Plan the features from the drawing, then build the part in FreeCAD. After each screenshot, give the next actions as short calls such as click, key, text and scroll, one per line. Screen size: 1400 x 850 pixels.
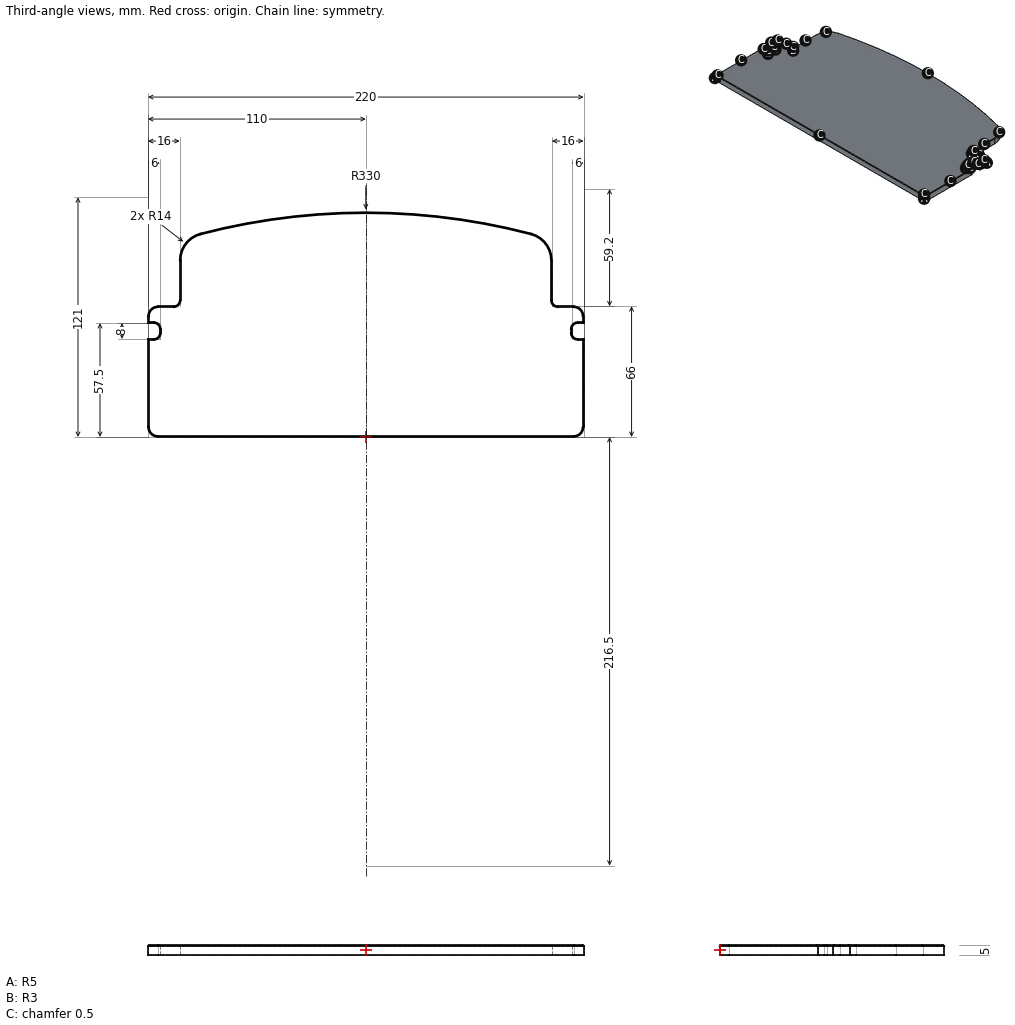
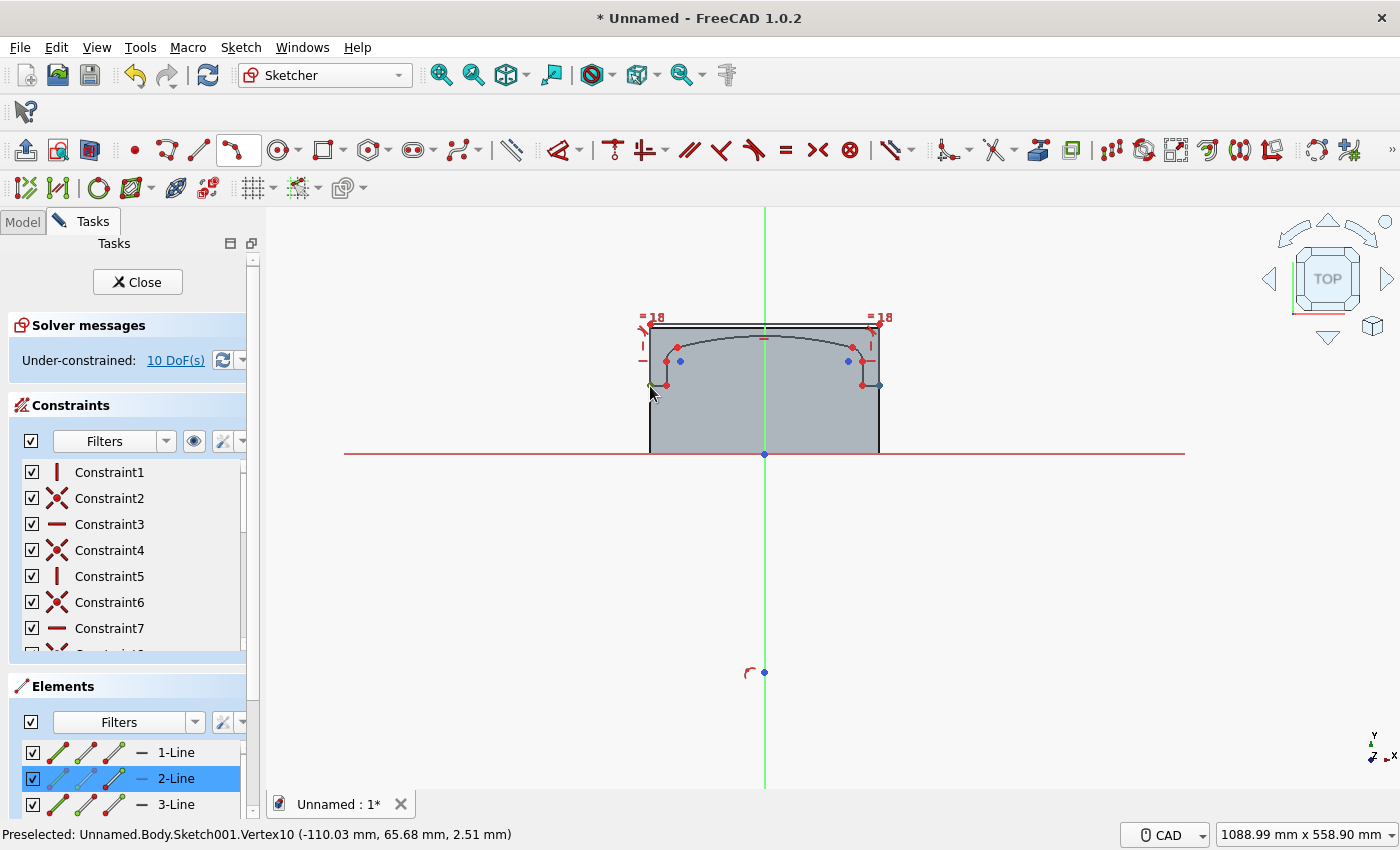
click(765, 723)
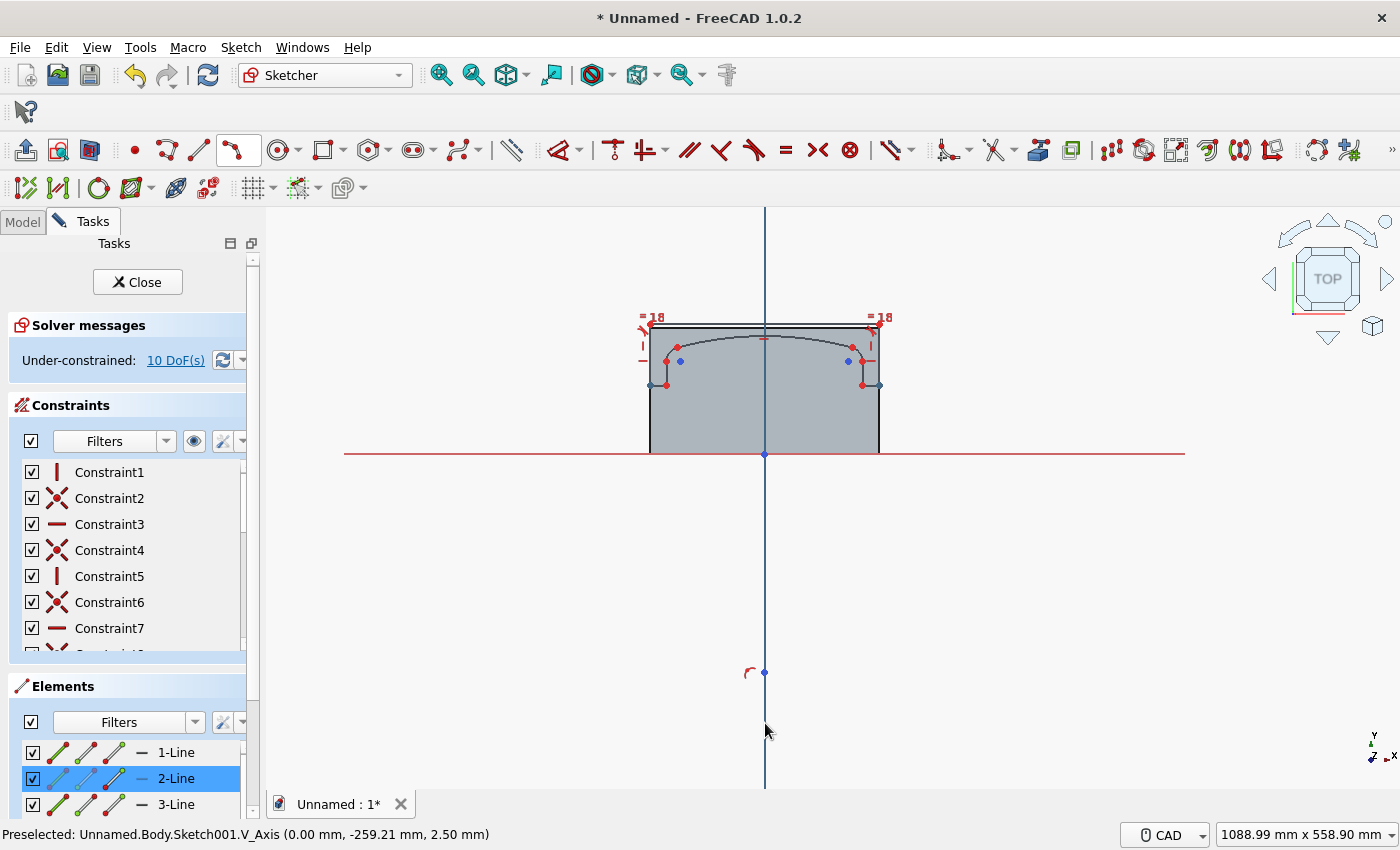
key(s)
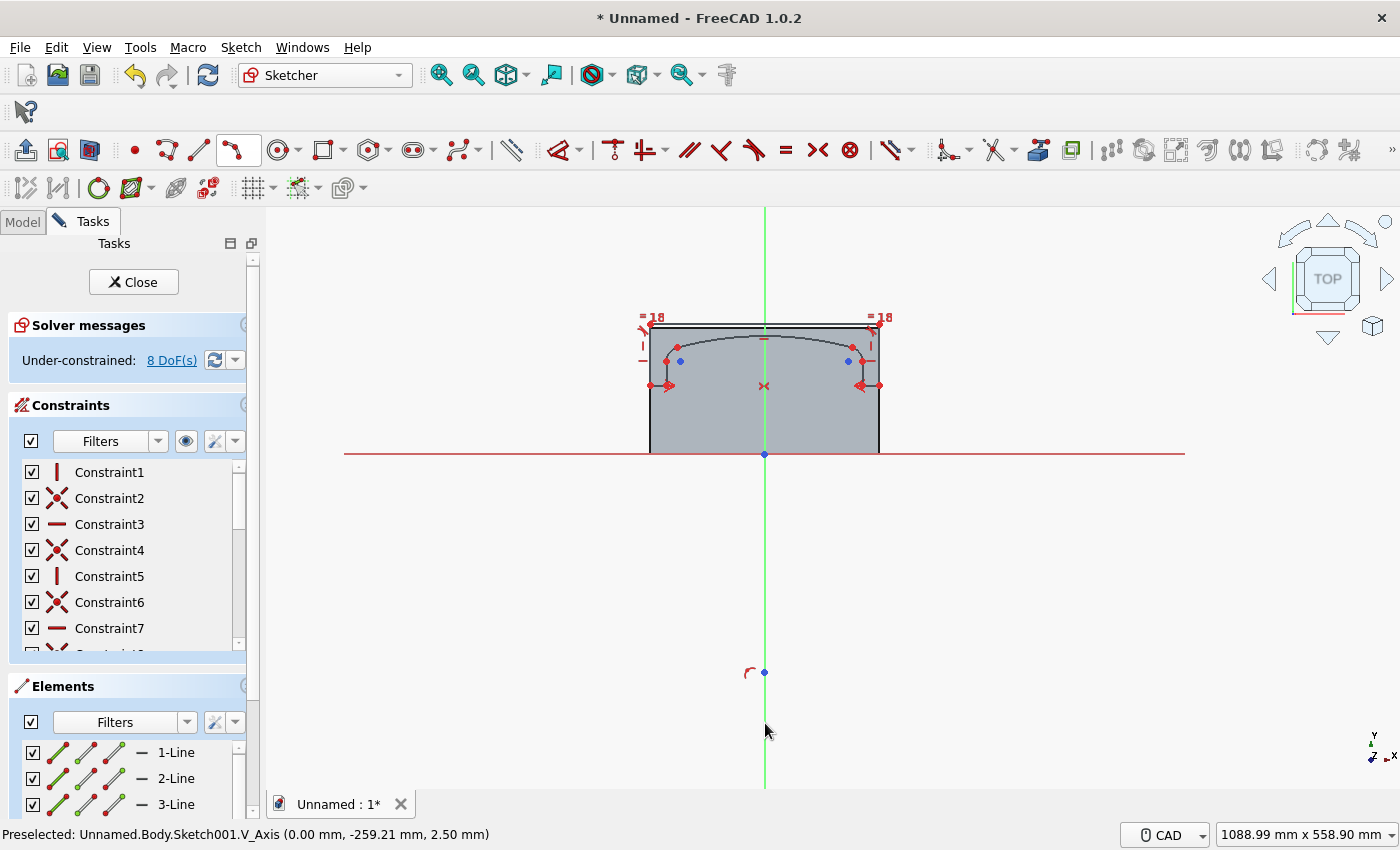
key(d)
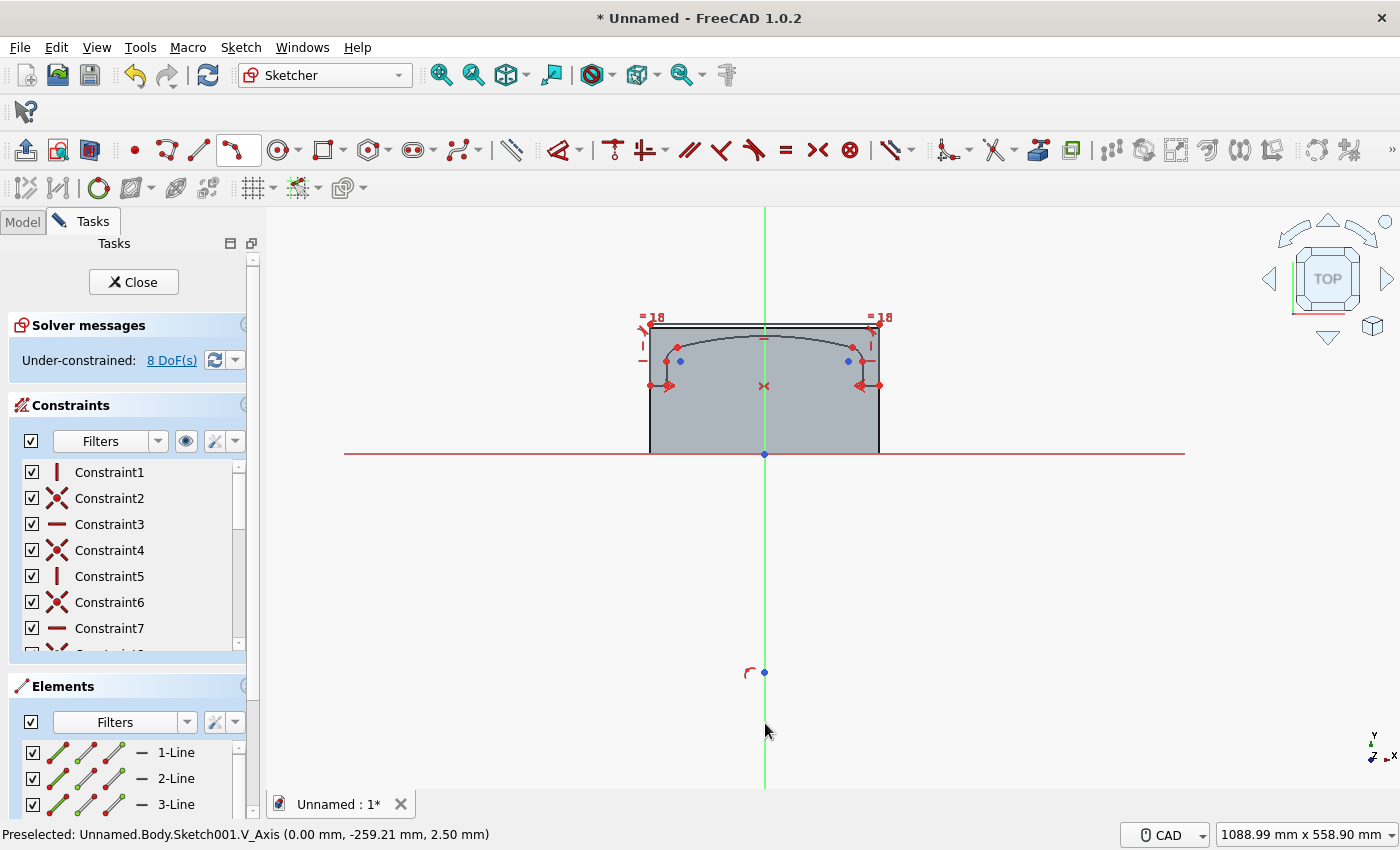
scroll(669, 353, up, 6)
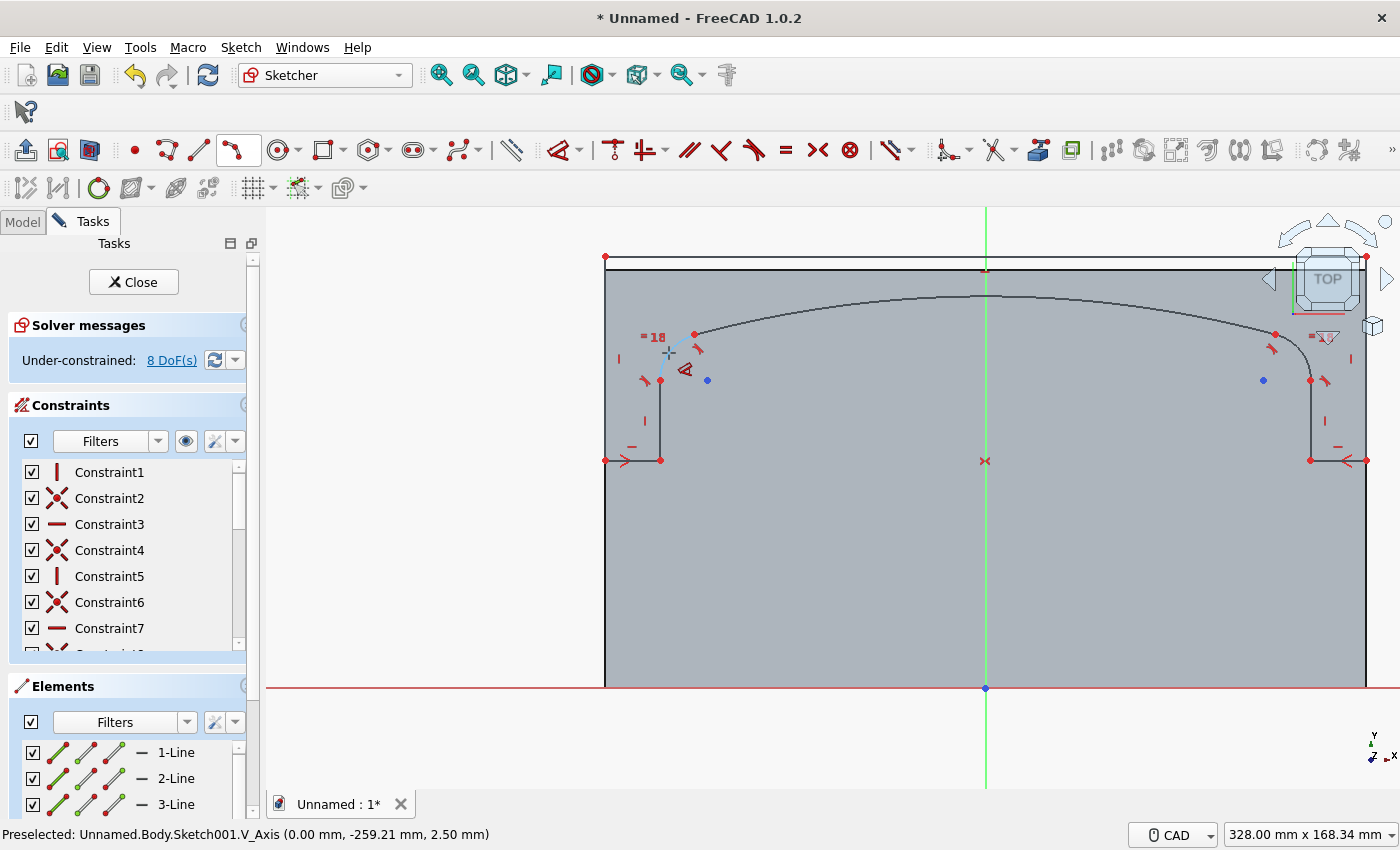
click(670, 352)
click(645, 333)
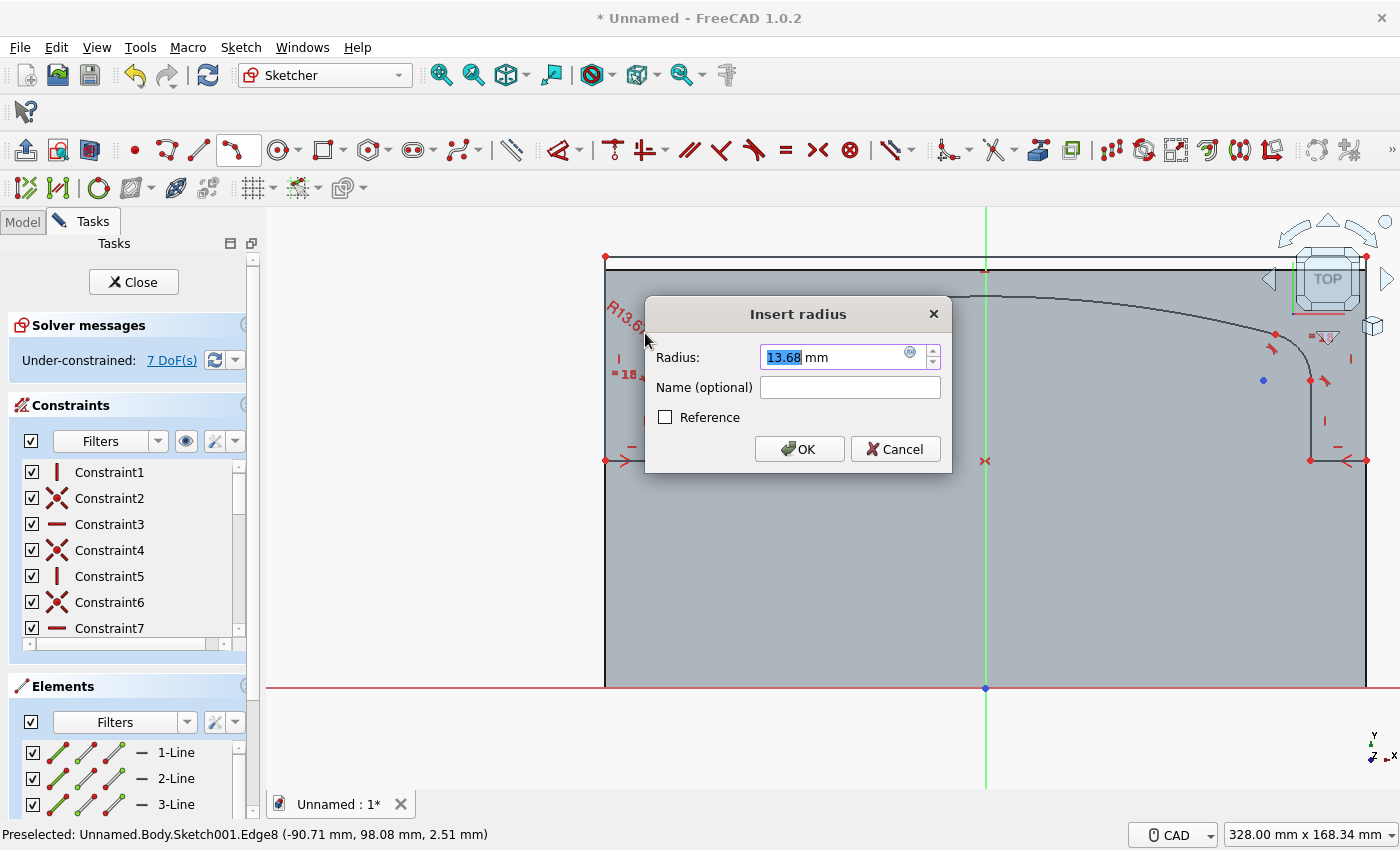
text(14)
key(Return)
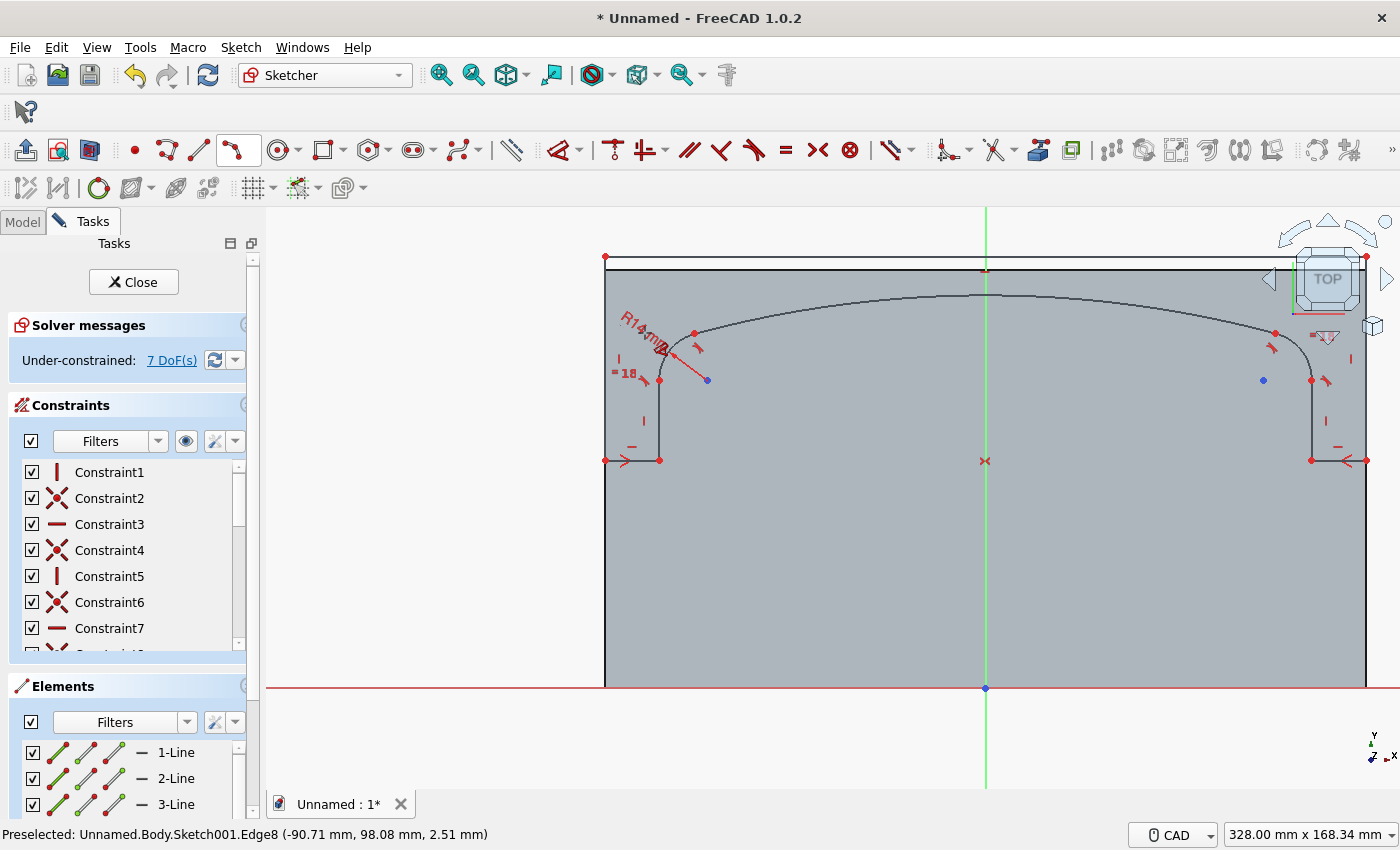
click(1103, 302)
click(1106, 270)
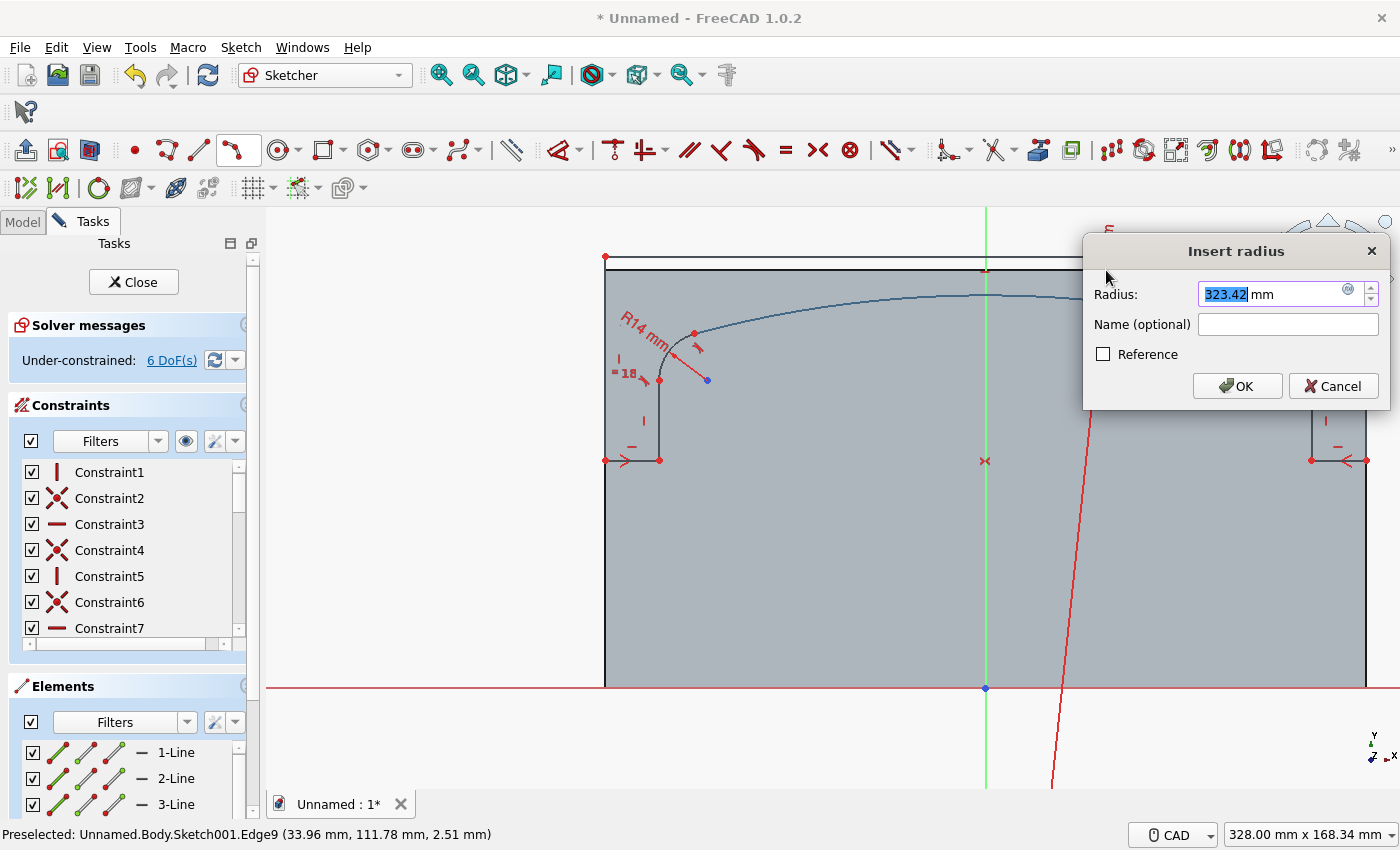
text(330)
key(Return)